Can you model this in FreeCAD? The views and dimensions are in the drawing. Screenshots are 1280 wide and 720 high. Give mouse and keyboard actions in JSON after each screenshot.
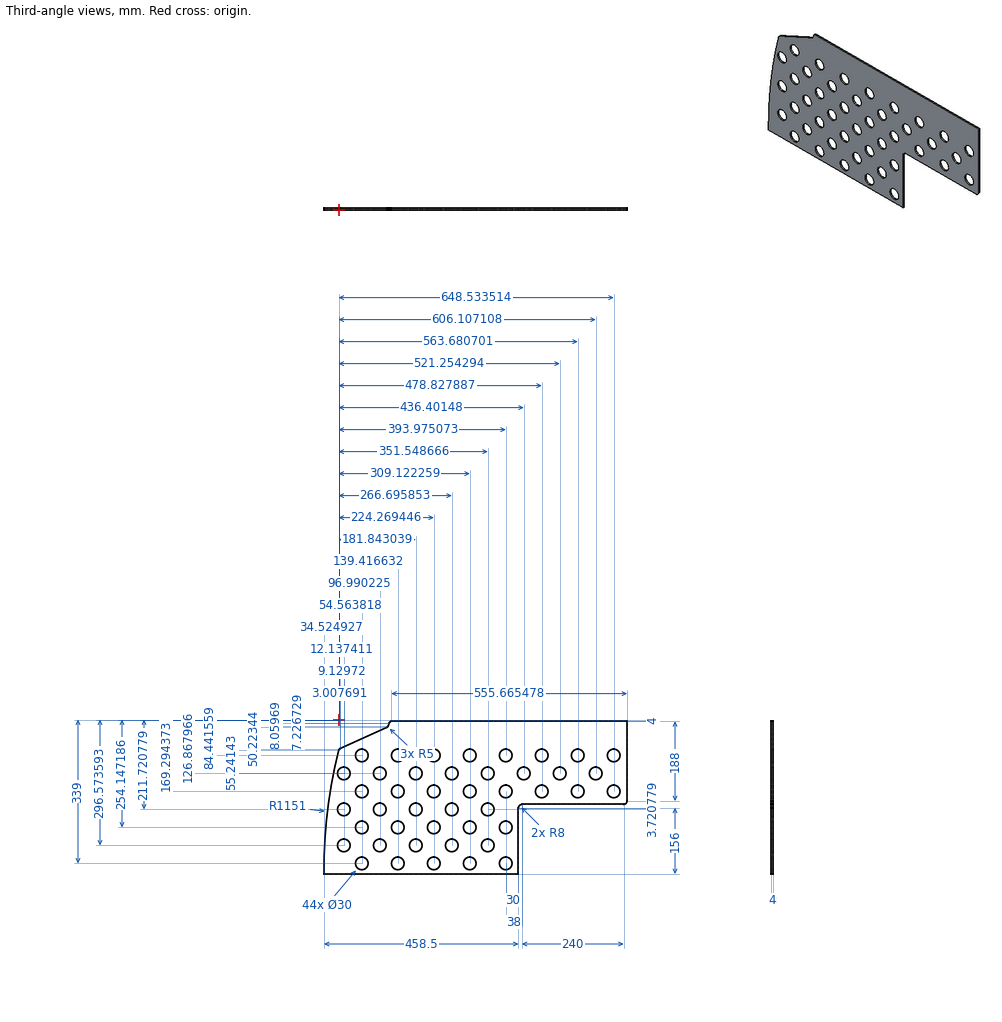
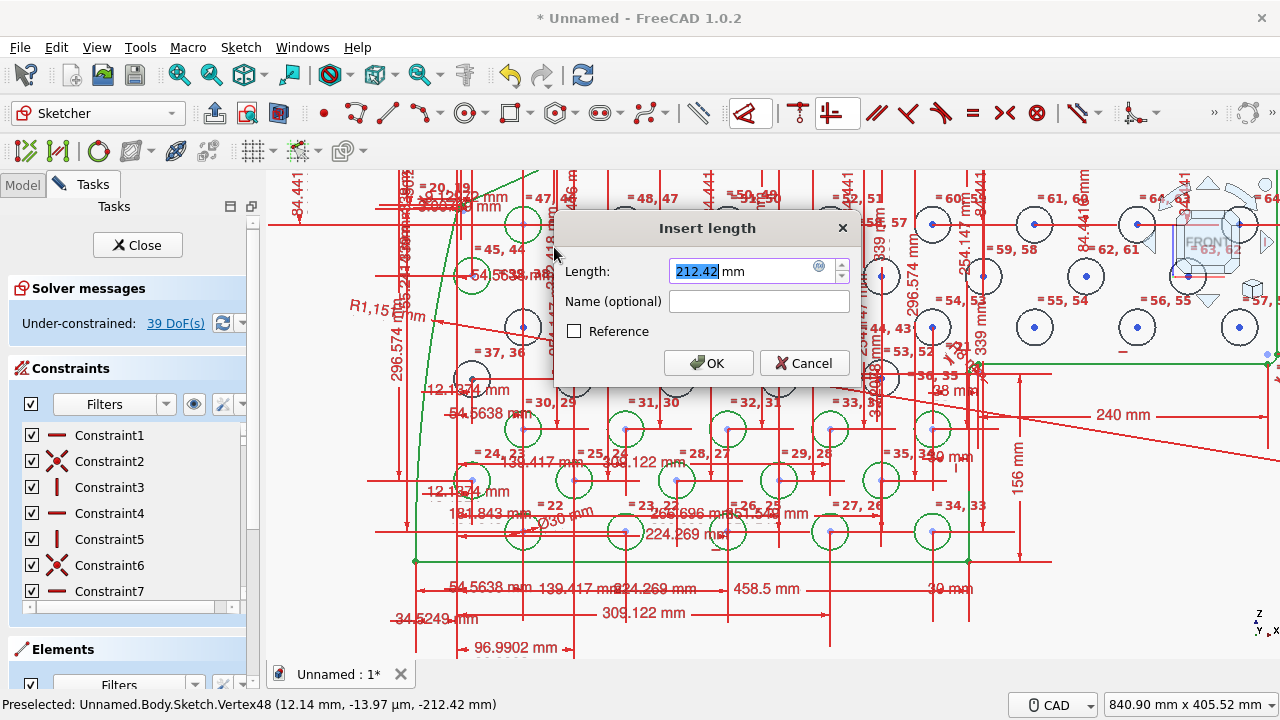
{"action": "type", "text": "211.720779"}
{"action": "key", "text": "Return"}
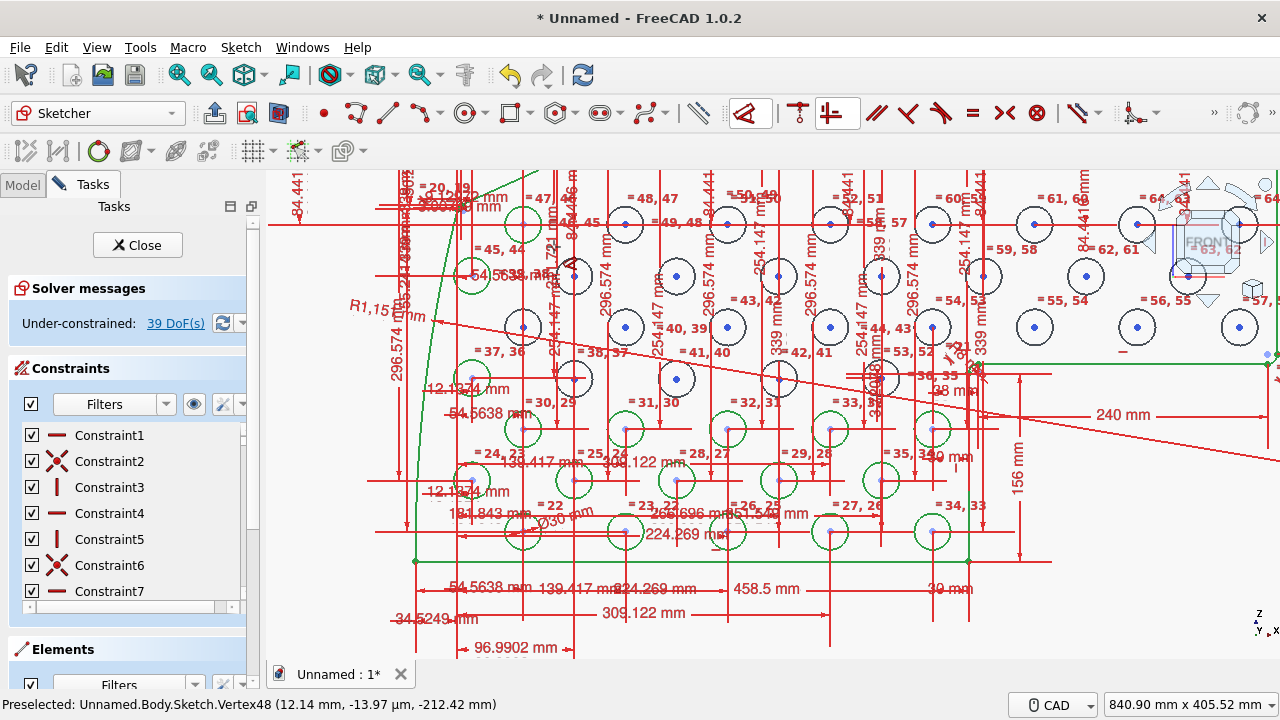
{"action": "left_click", "coordinate": [574, 379]}
{"action": "left_click", "coordinate": [656, 247]}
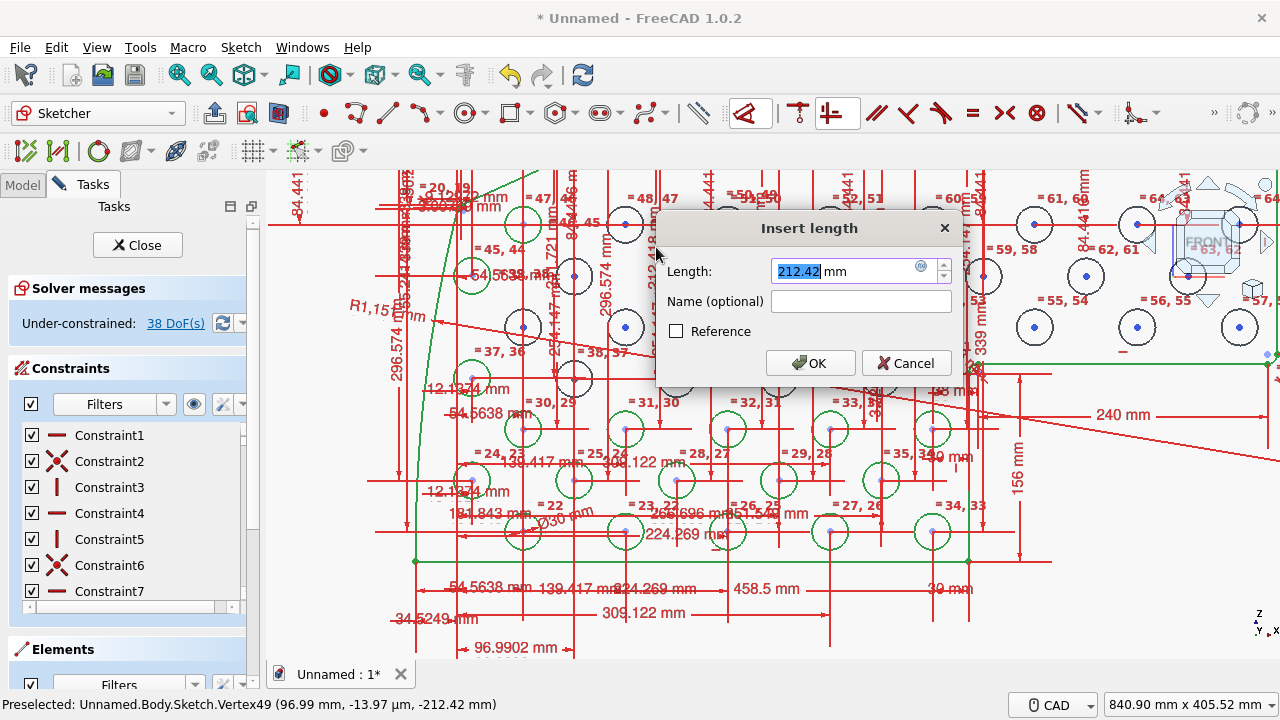
{"action": "type", "text": "211.720779"}
{"action": "key", "text": "Return"}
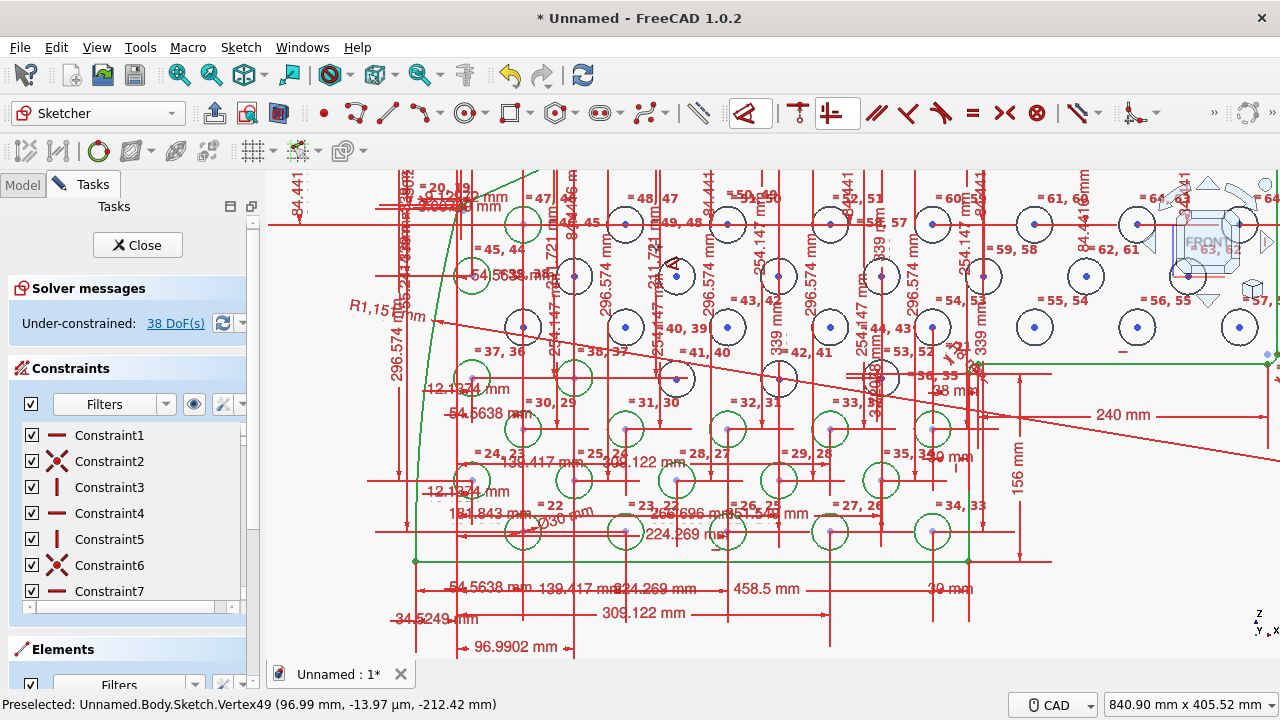
{"action": "left_click", "coordinate": [523, 327]}
{"action": "left_click", "coordinate": [327, 263]}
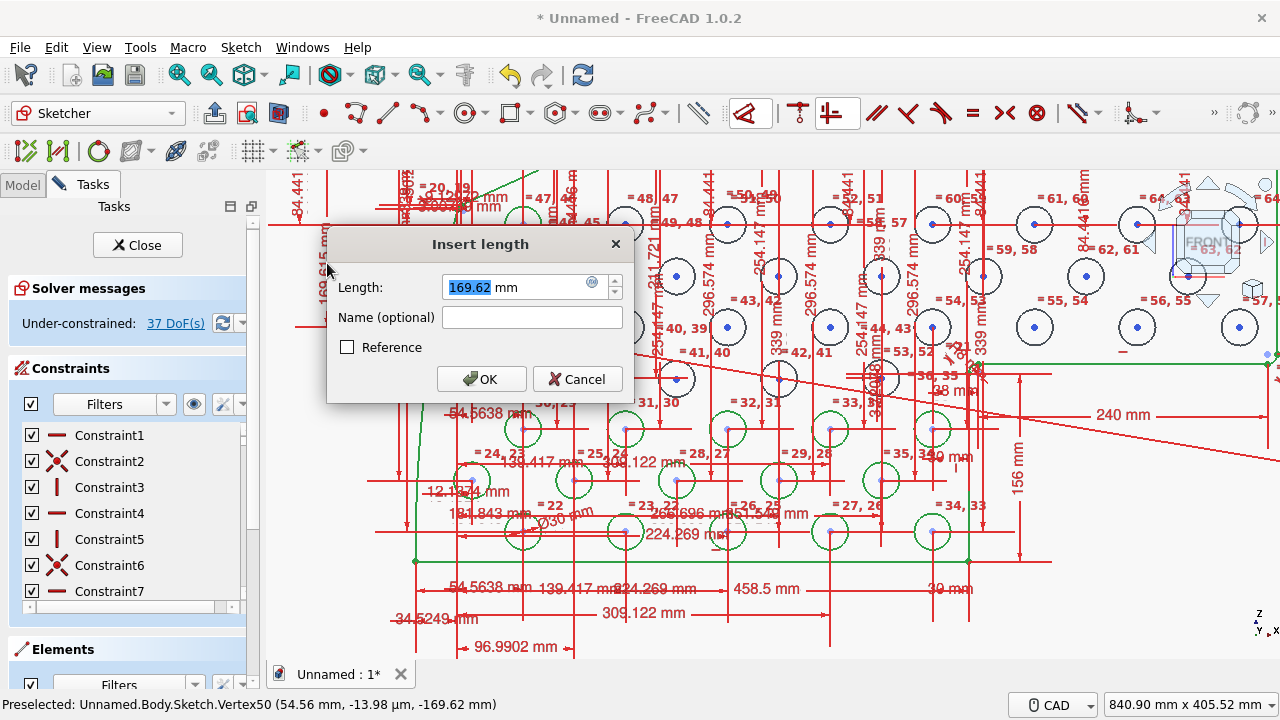
{"action": "type", "text": "169.294373"}
{"action": "key", "text": "Return"}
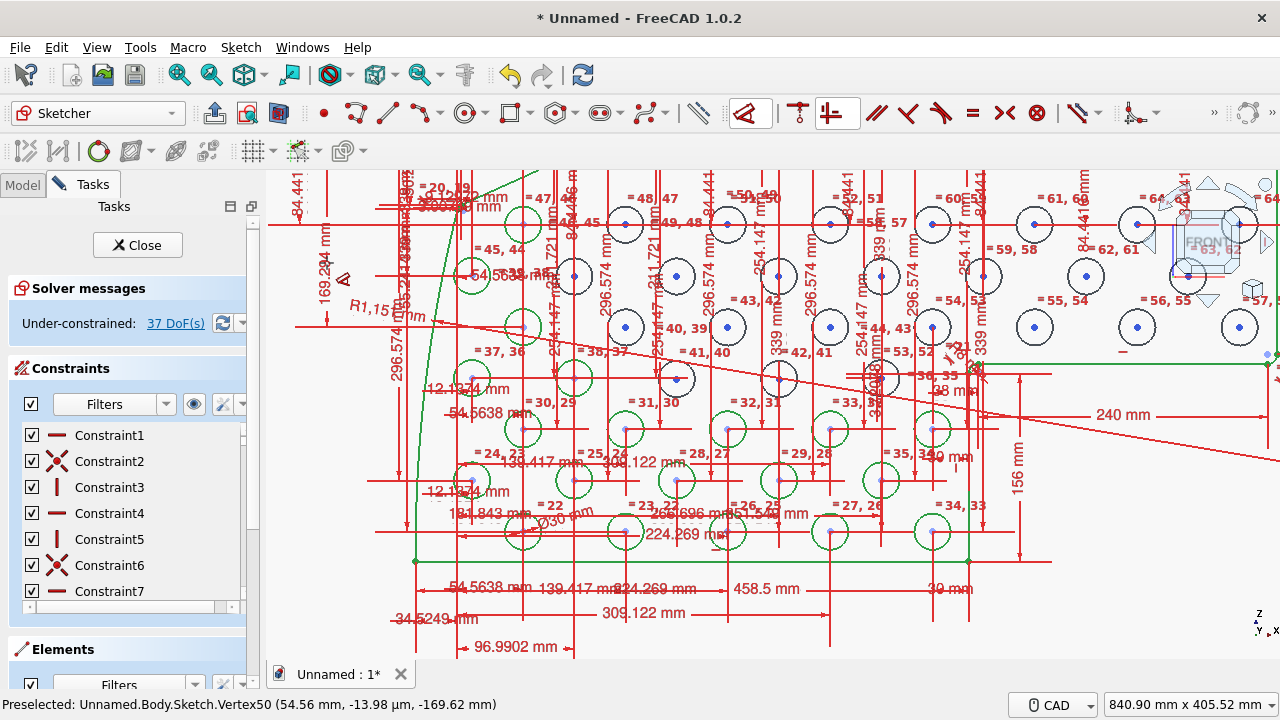
{"action": "left_click", "coordinate": [626, 327]}
{"action": "left_click", "coordinate": [542, 361]}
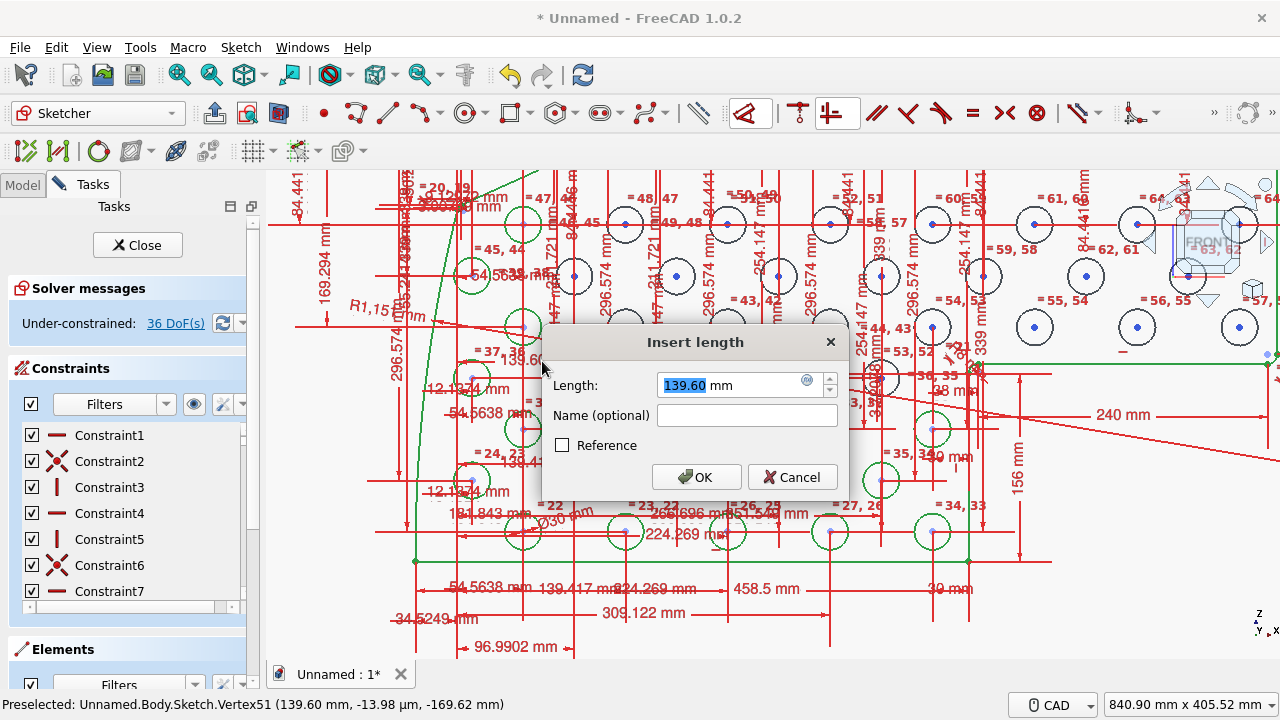
{"action": "type", "text": "139.416632"}
{"action": "key", "text": "Return"}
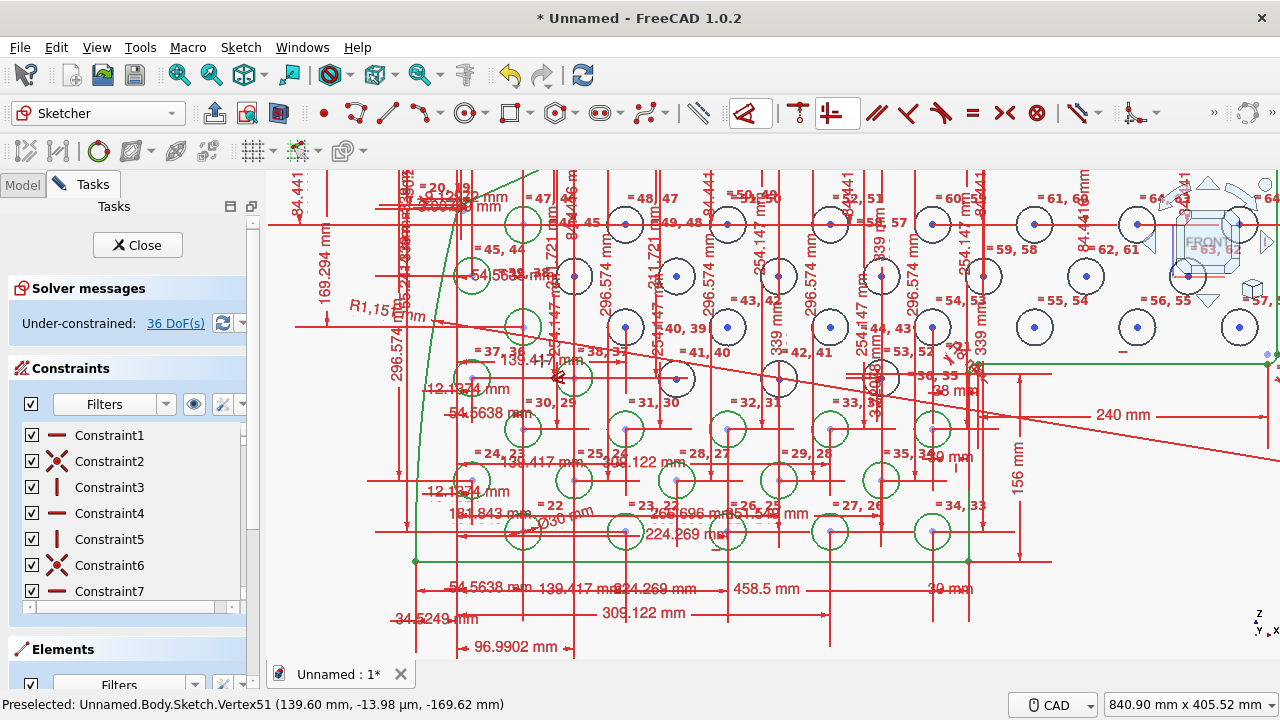
{"action": "left_click", "coordinate": [626, 327]}
{"action": "left_click", "coordinate": [660, 217]}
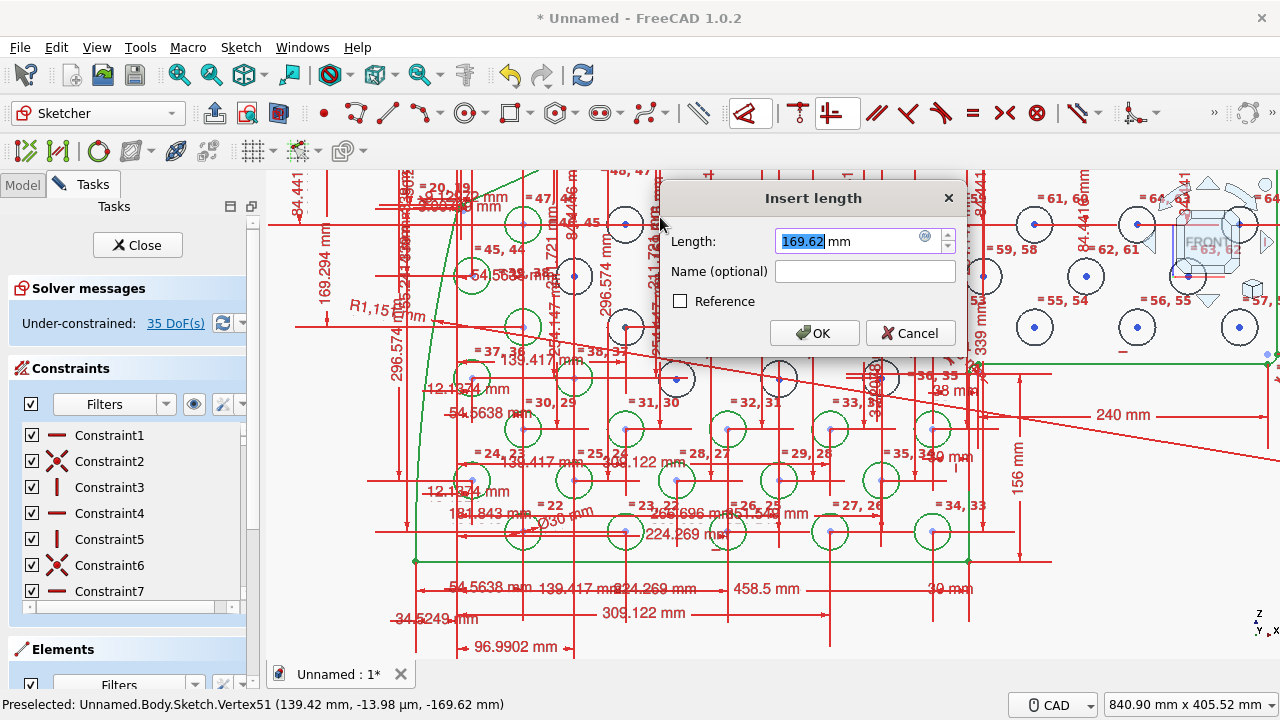
{"action": "type", "text": "169.294373"}
{"action": "key", "text": "Return"}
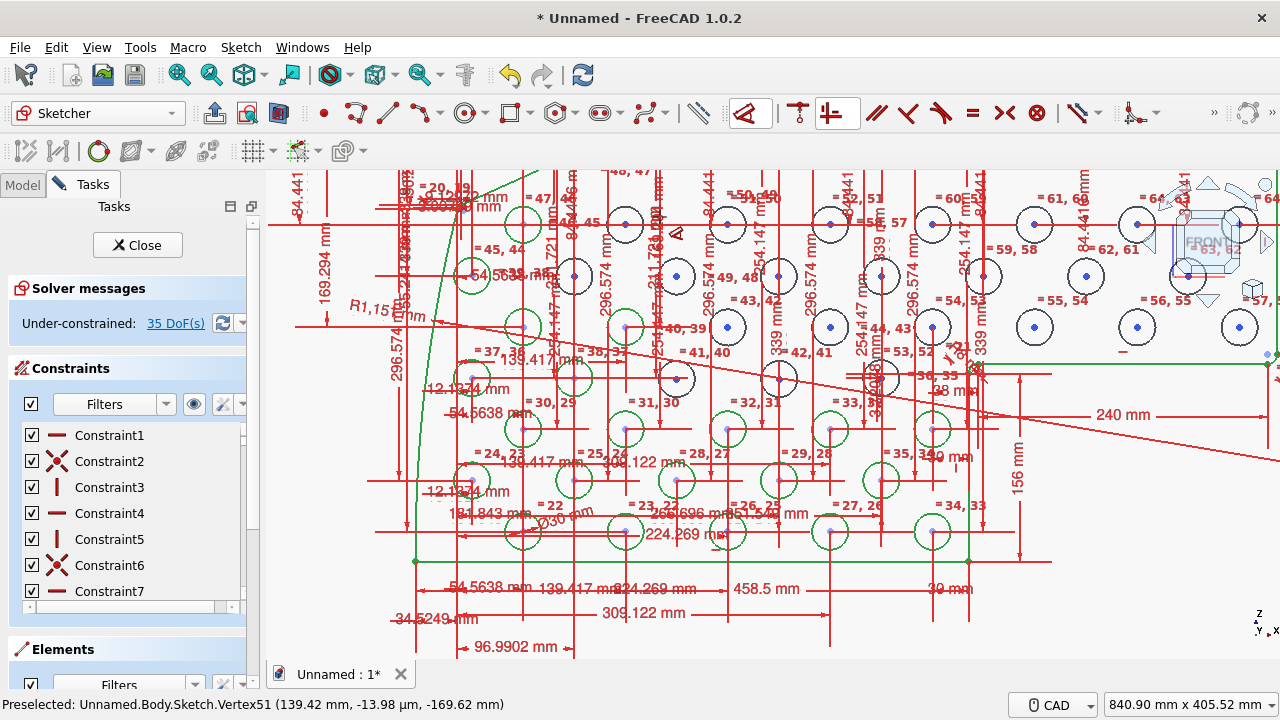
{"action": "left_click", "coordinate": [677, 379]}
{"action": "left_click", "coordinate": [567, 413]}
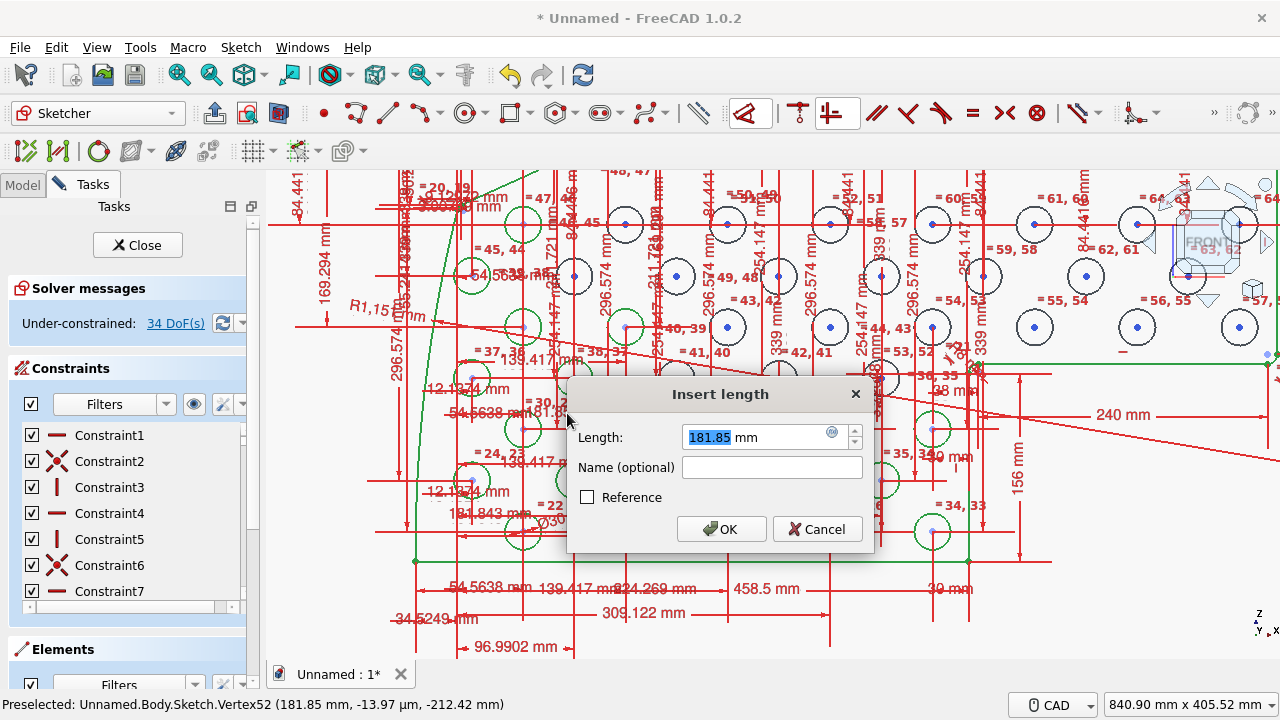
{"action": "type", "text": "181.843039"}
{"action": "key", "text": "Return"}